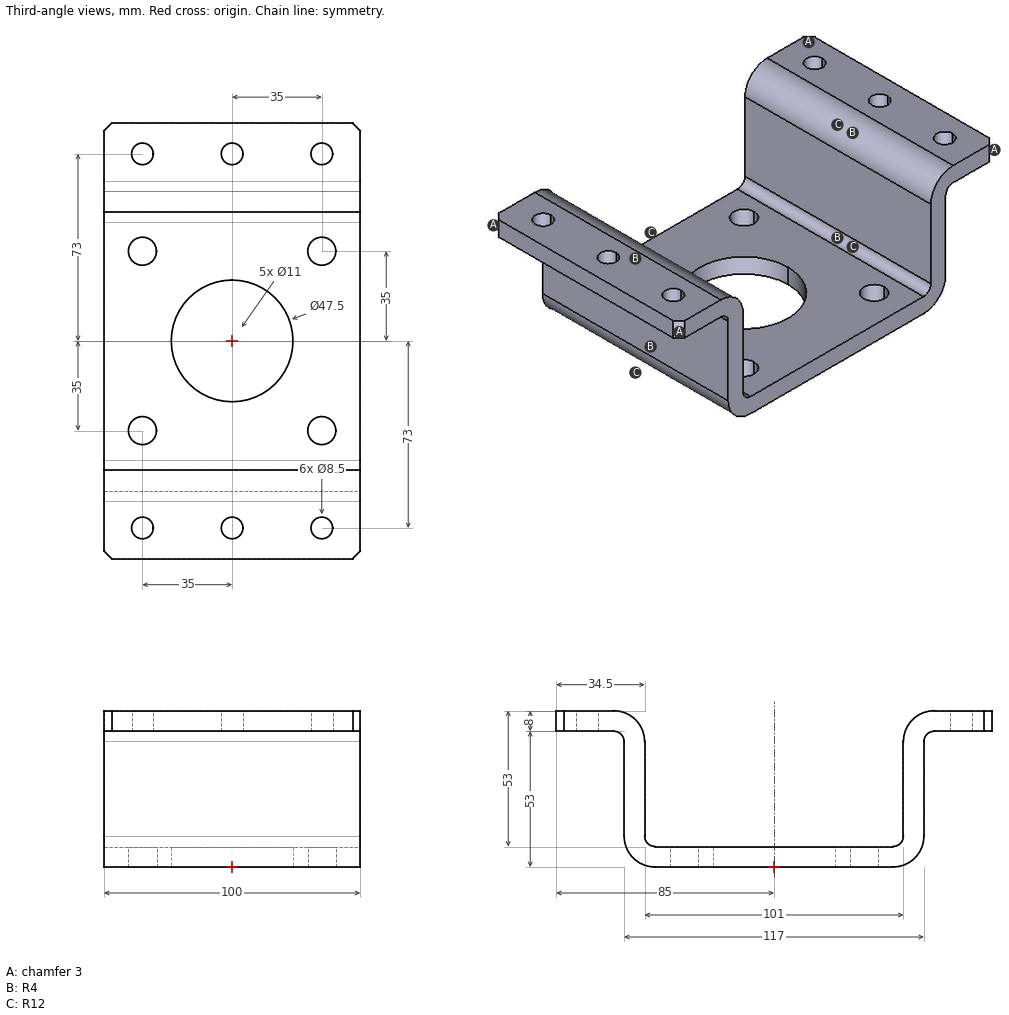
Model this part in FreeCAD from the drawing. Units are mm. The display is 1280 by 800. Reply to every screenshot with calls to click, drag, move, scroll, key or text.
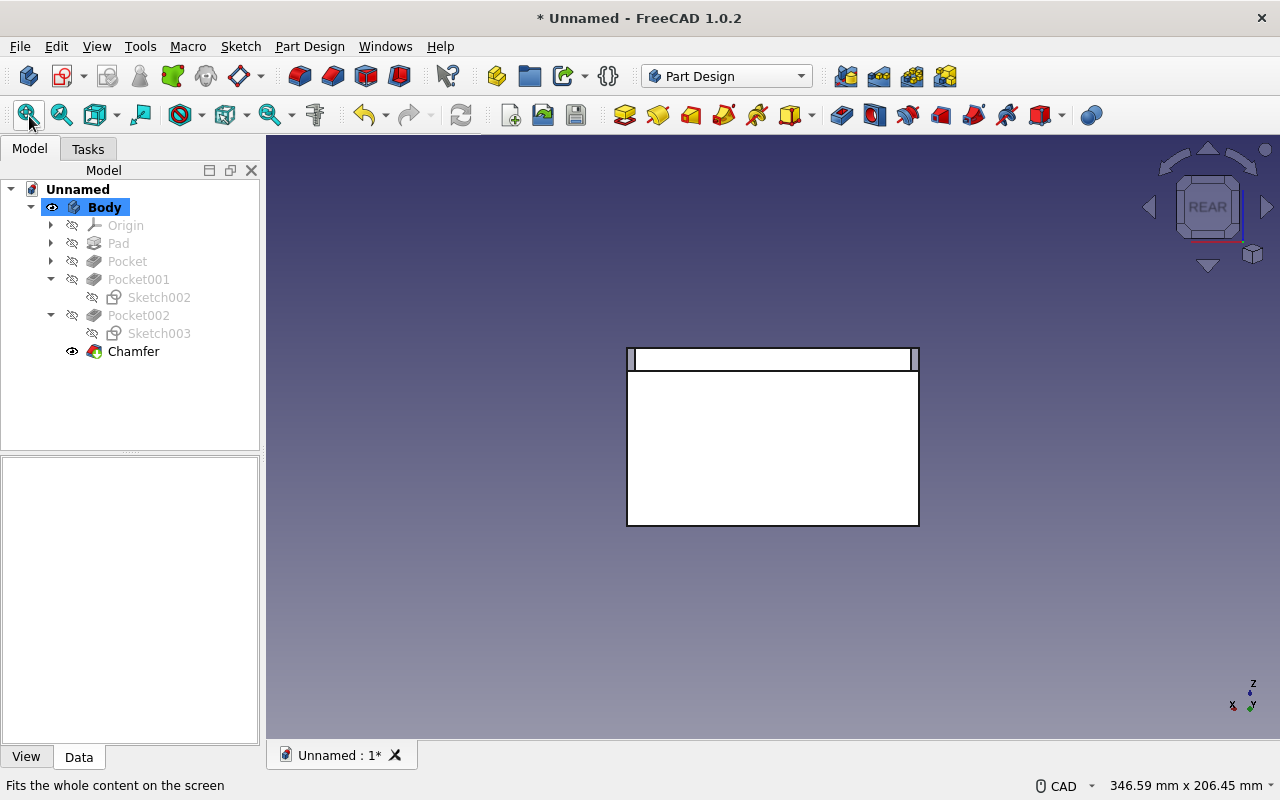
key(6)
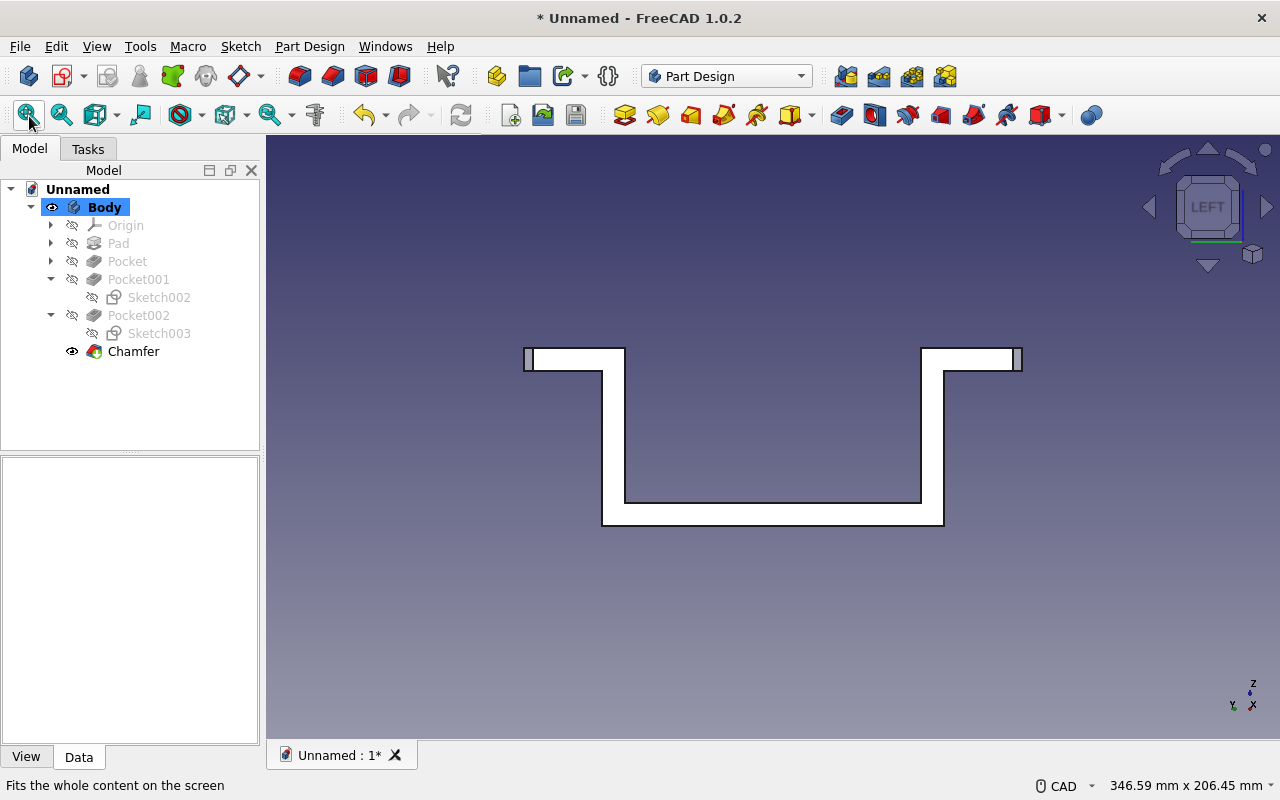
key(v)
key(3)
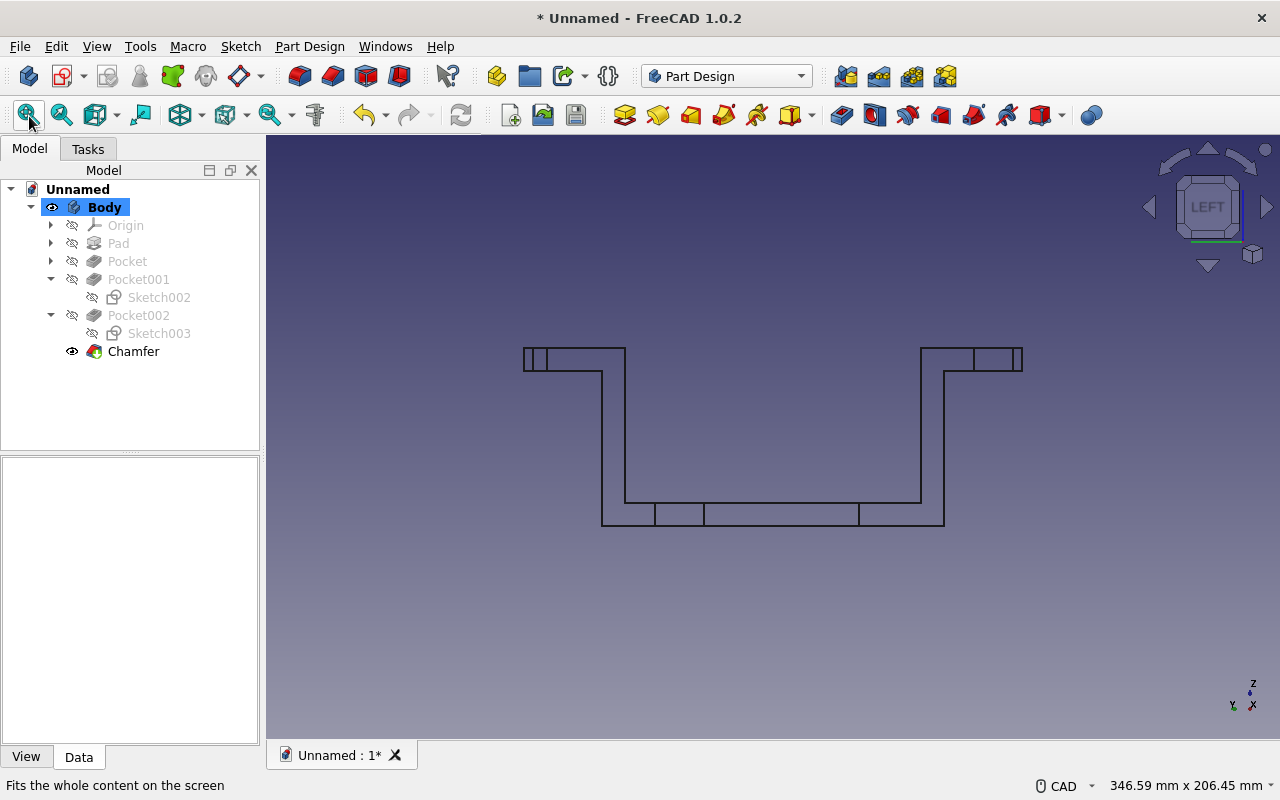
key(0)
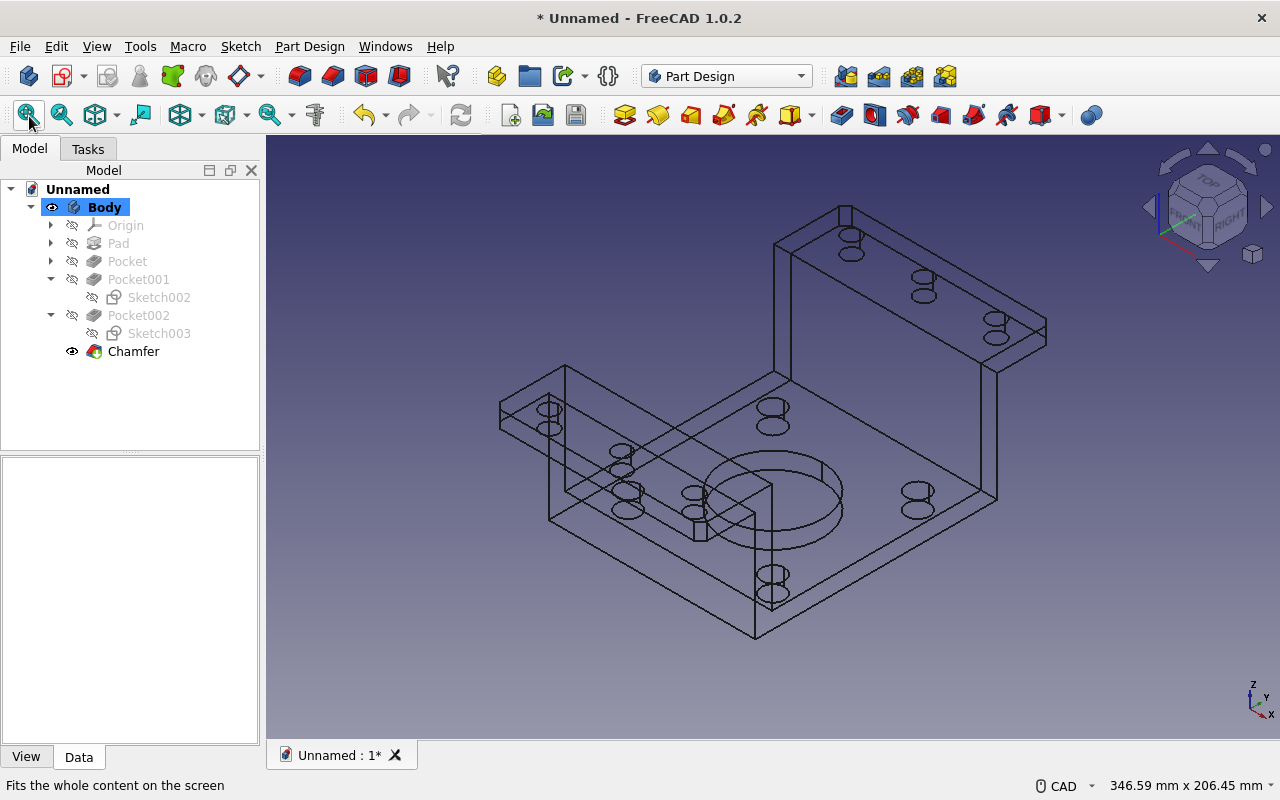
click(652, 452)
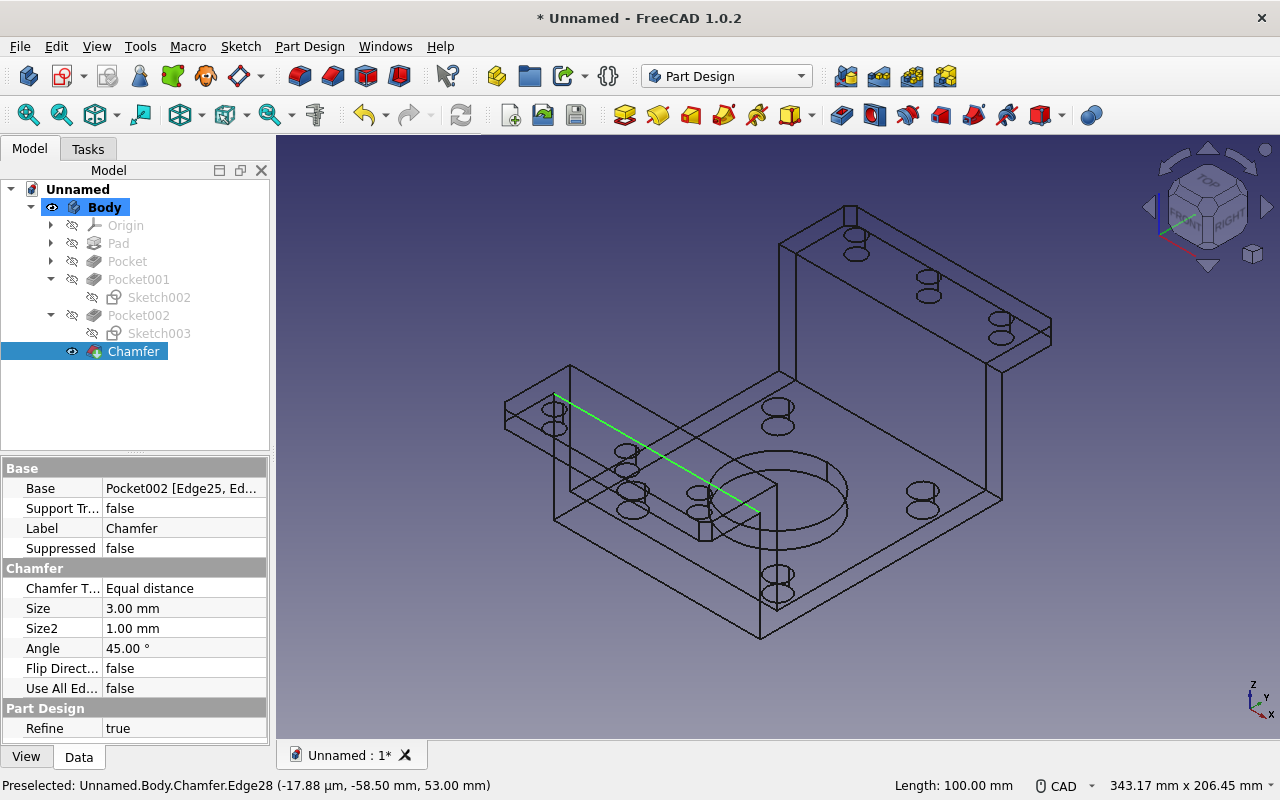
click(674, 550, ctrl)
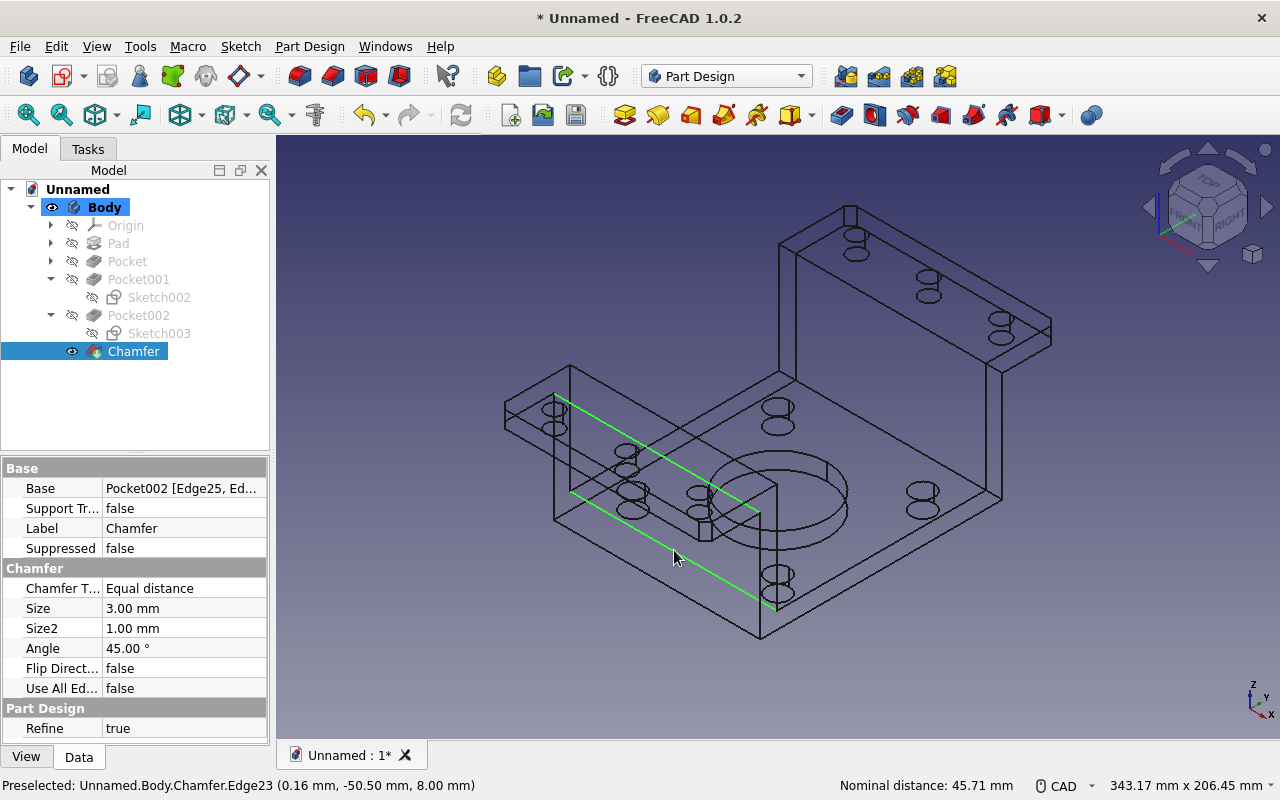
click(882, 429, ctrl)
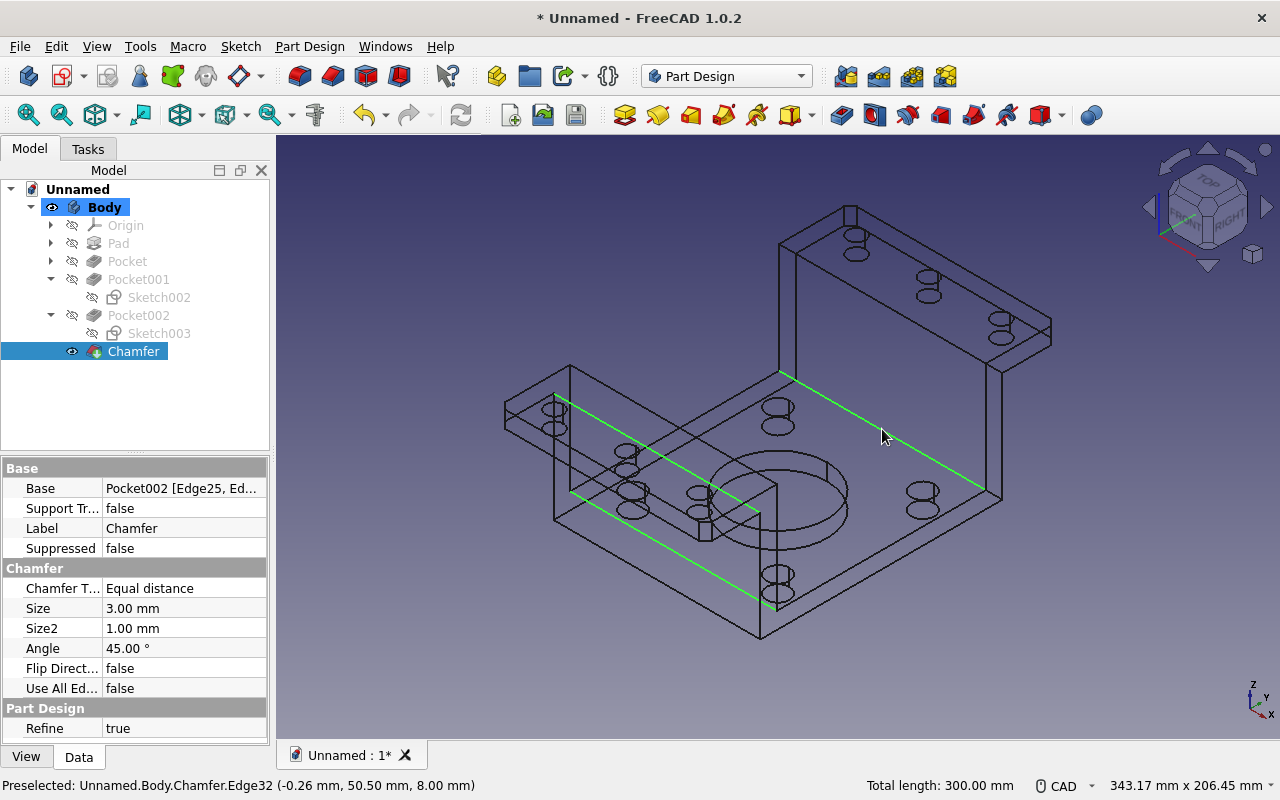
key(2)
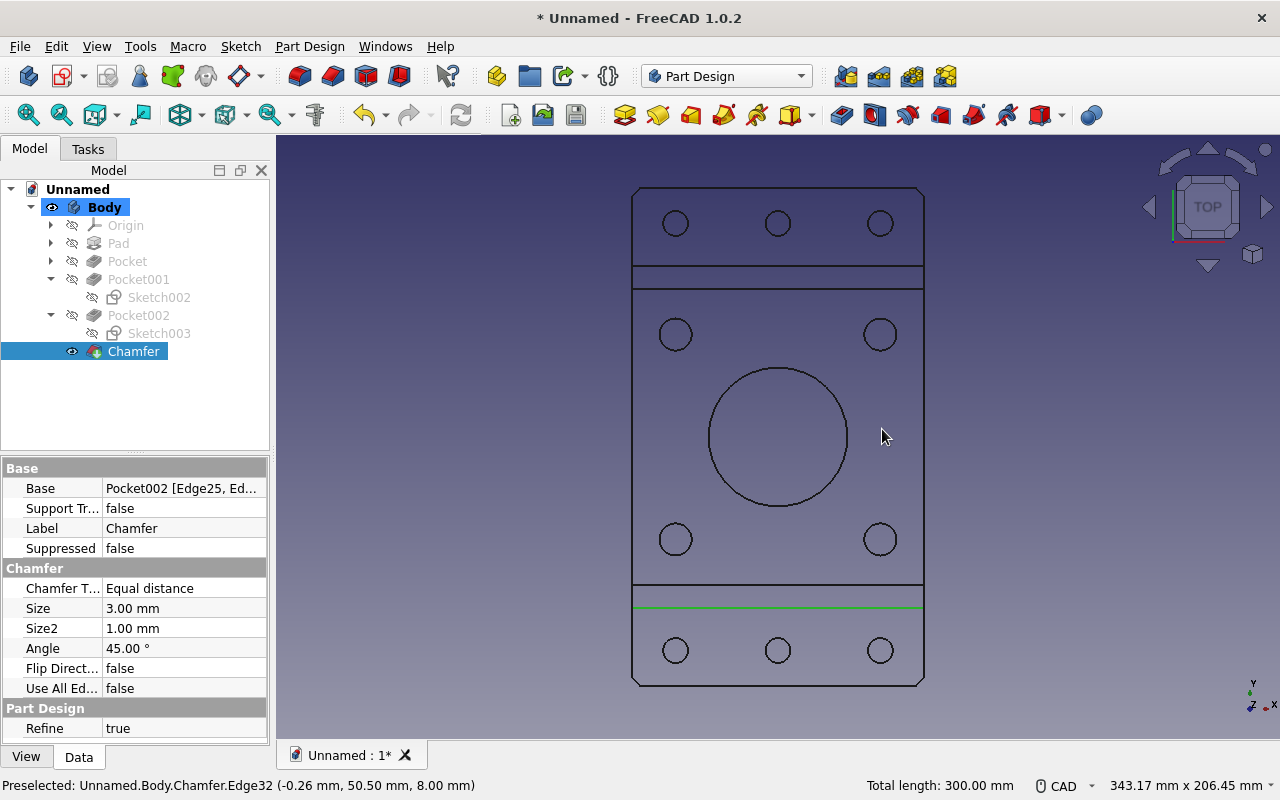
click(778, 265, ctrl)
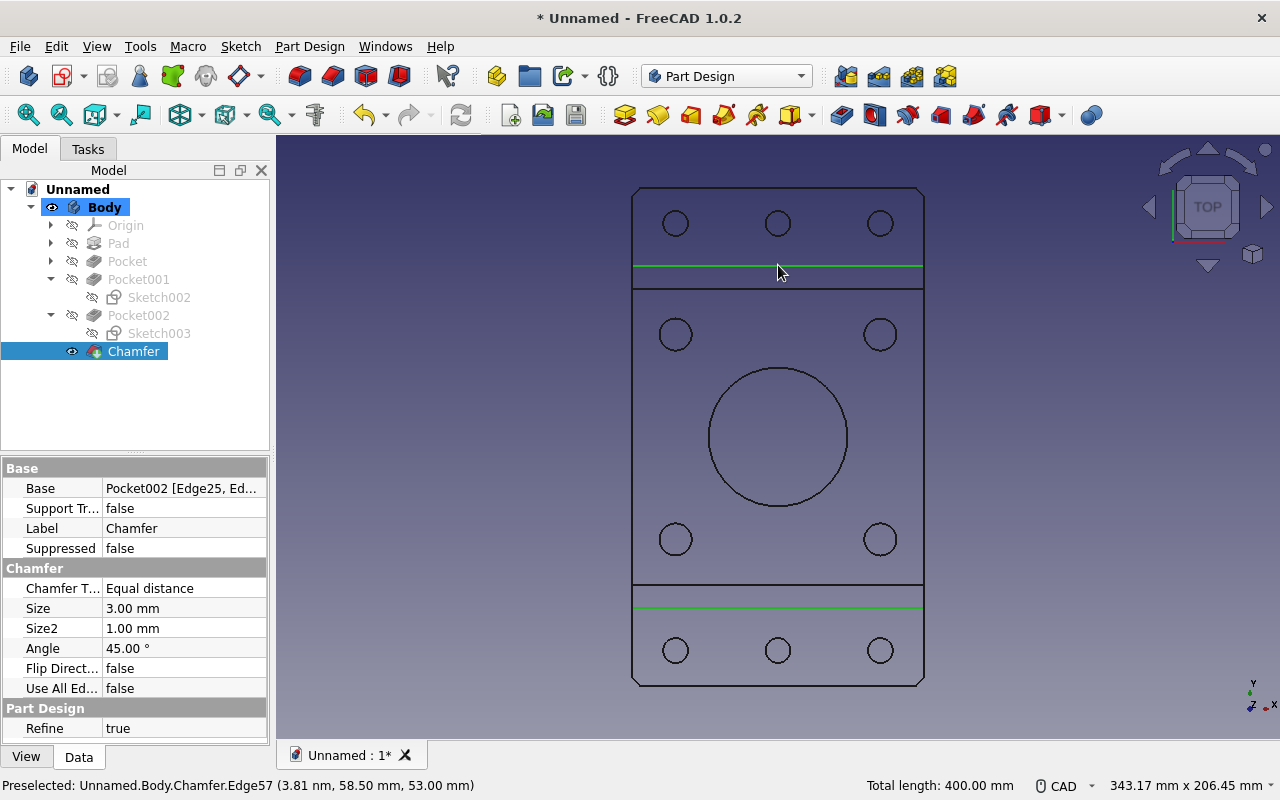
key(v)
key(1)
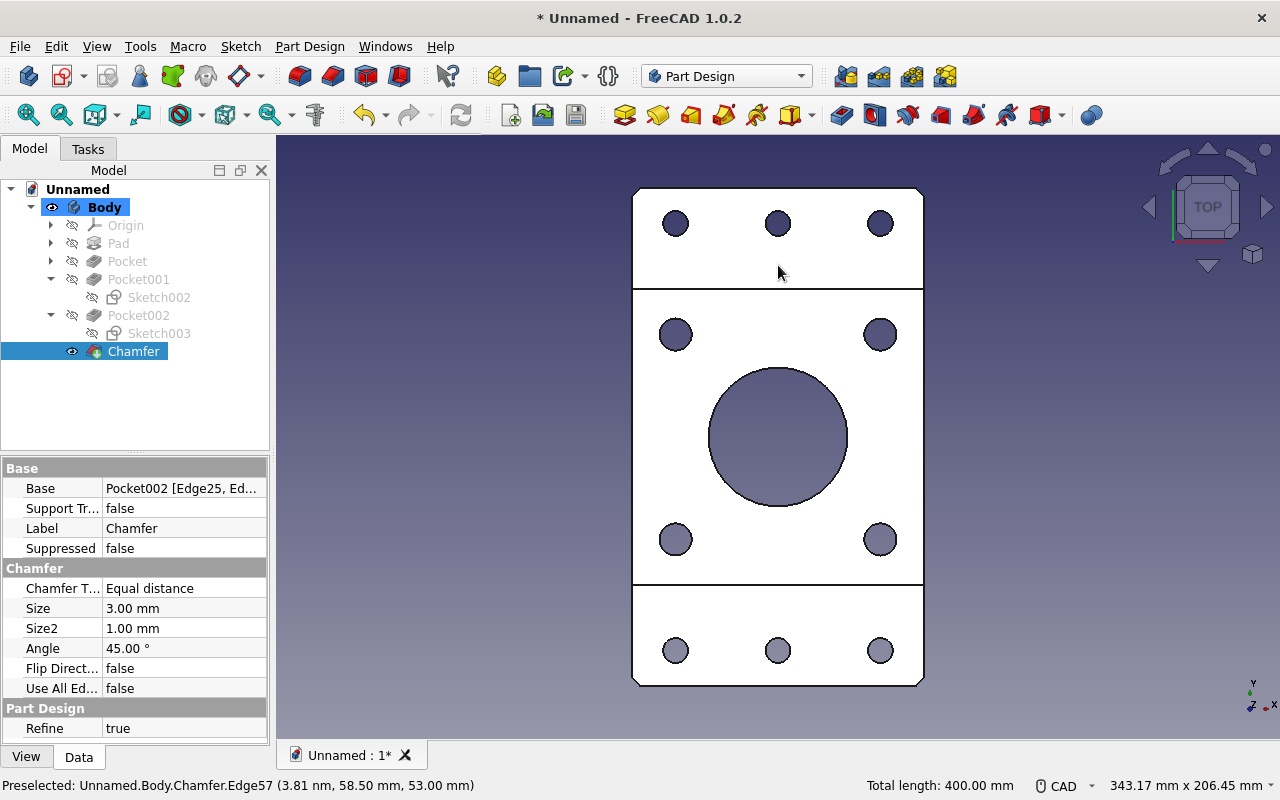
click(300, 76)